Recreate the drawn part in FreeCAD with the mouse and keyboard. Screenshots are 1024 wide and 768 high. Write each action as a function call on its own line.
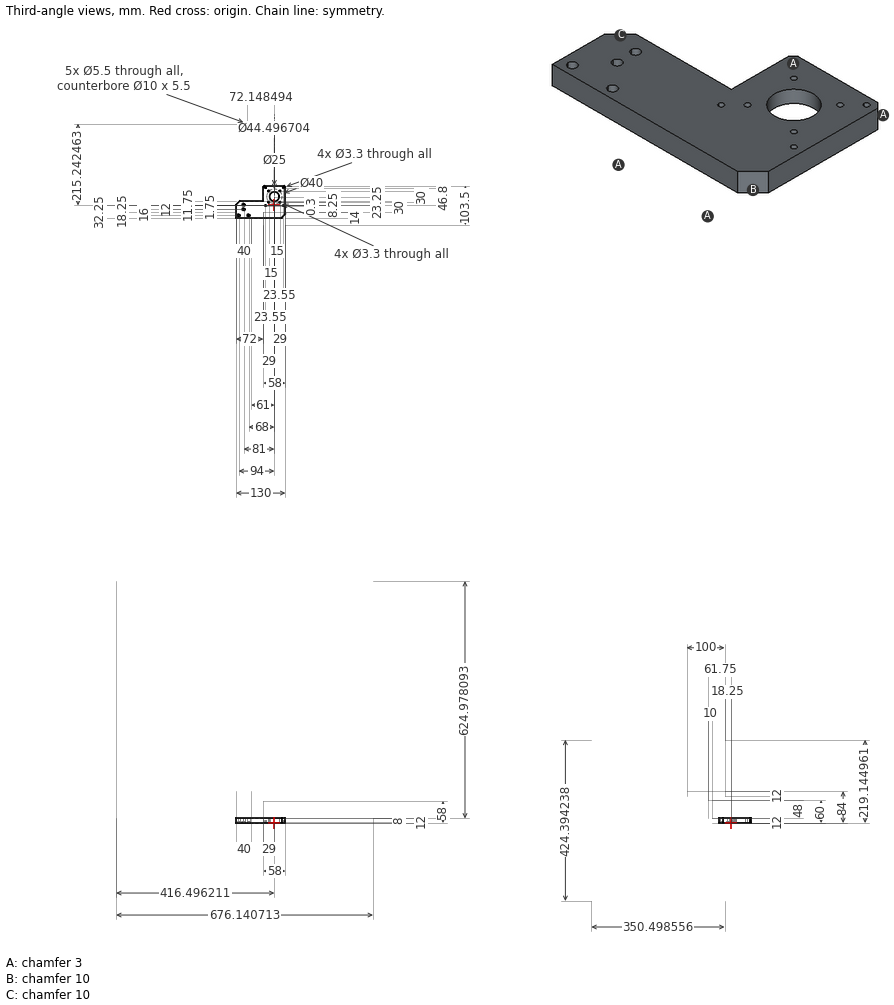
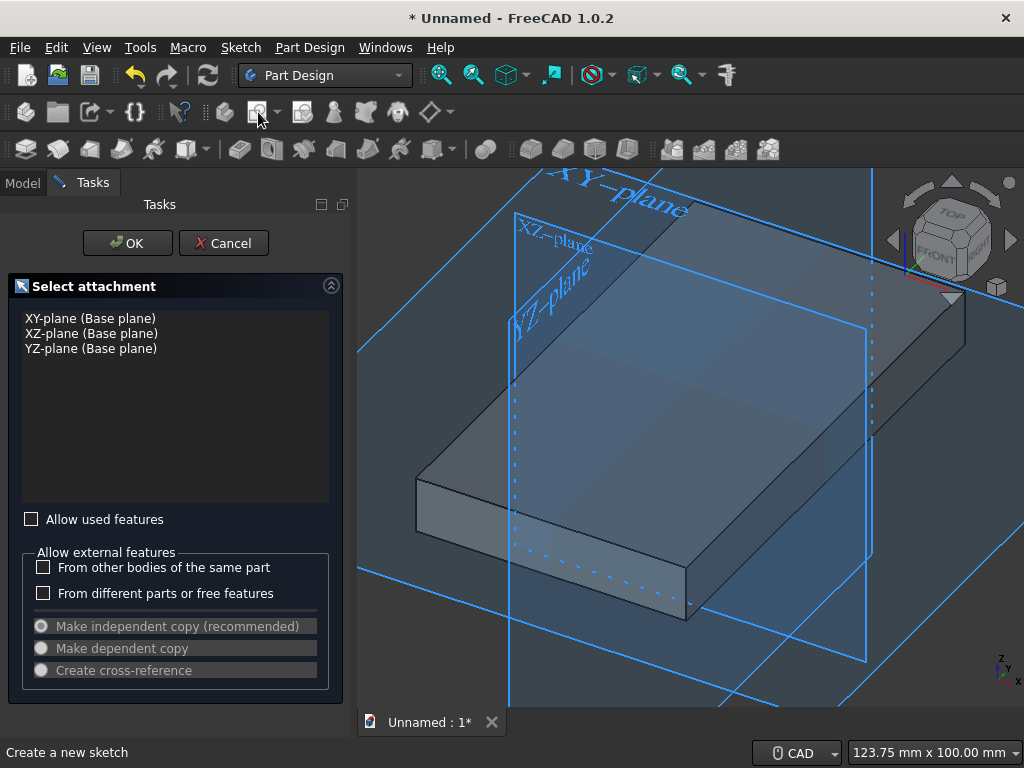
click(82, 318)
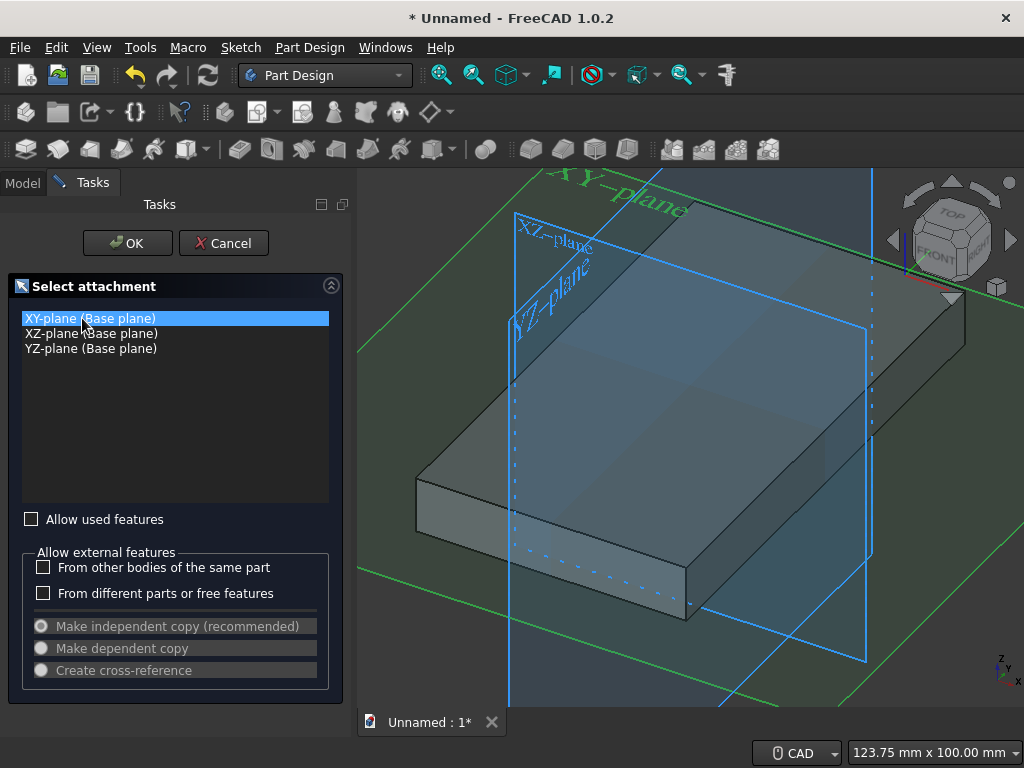
click(128, 243)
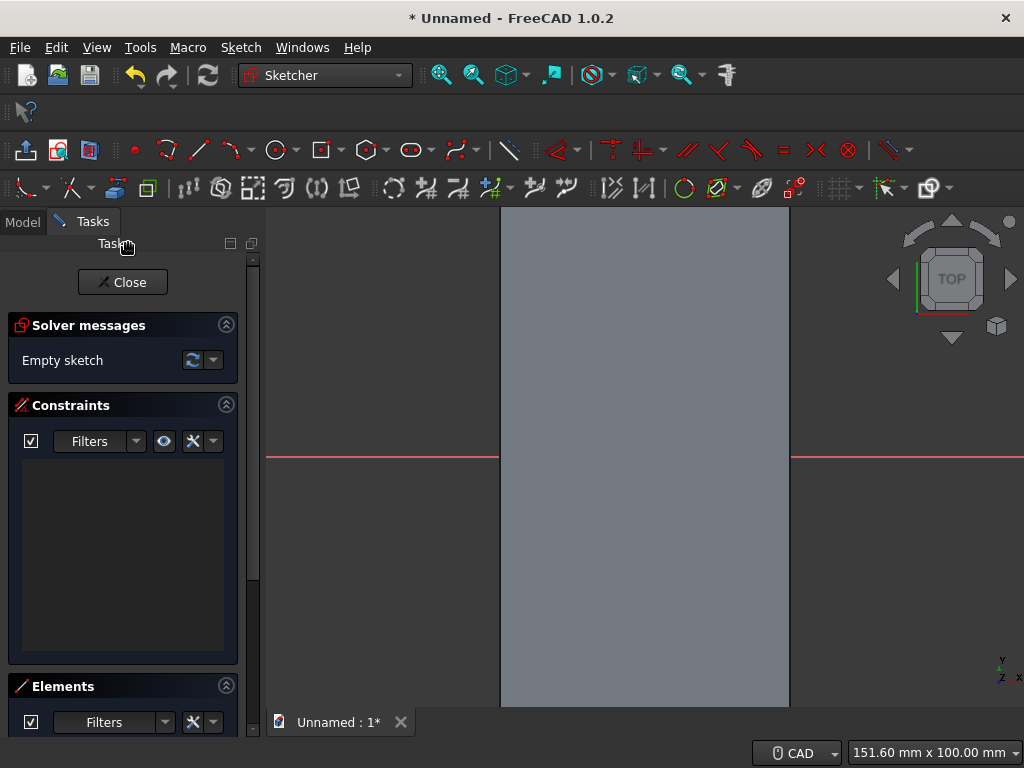
click(90, 150)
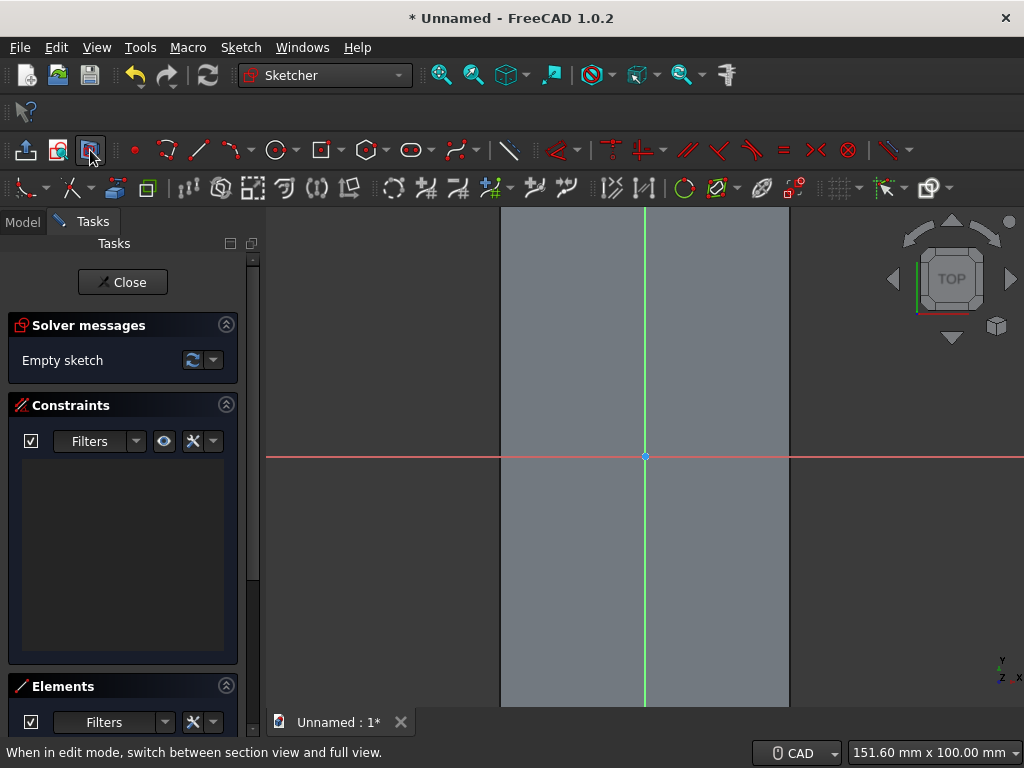
scroll(294, 679, down, 1)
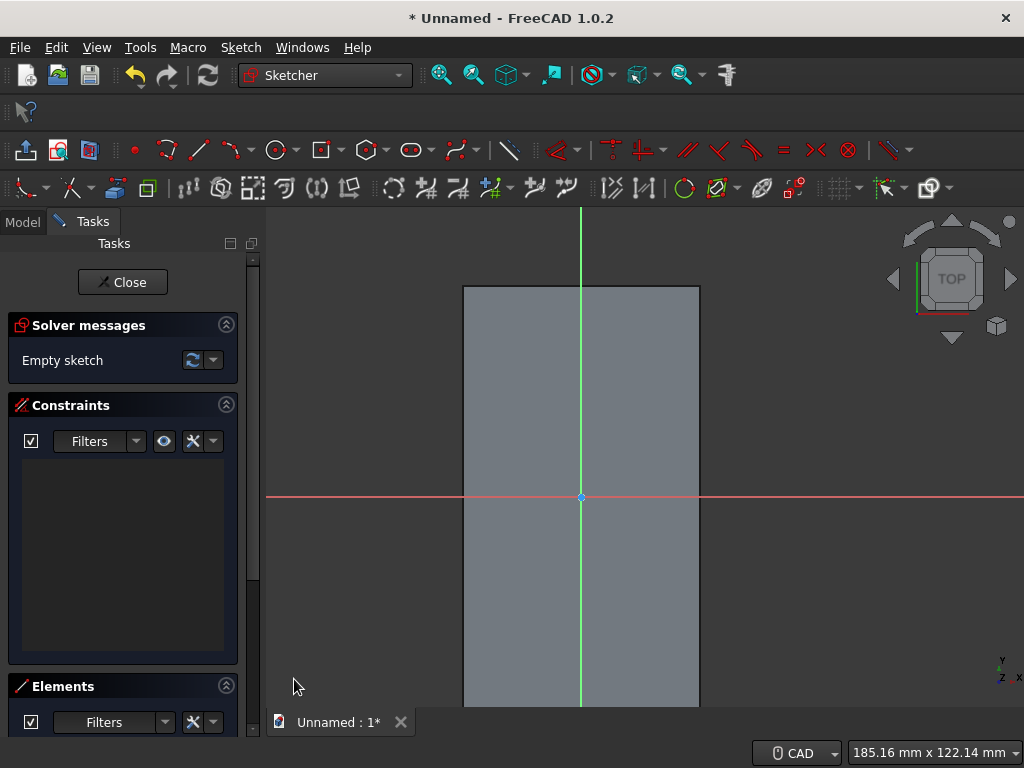
scroll(591, 291, up, 2)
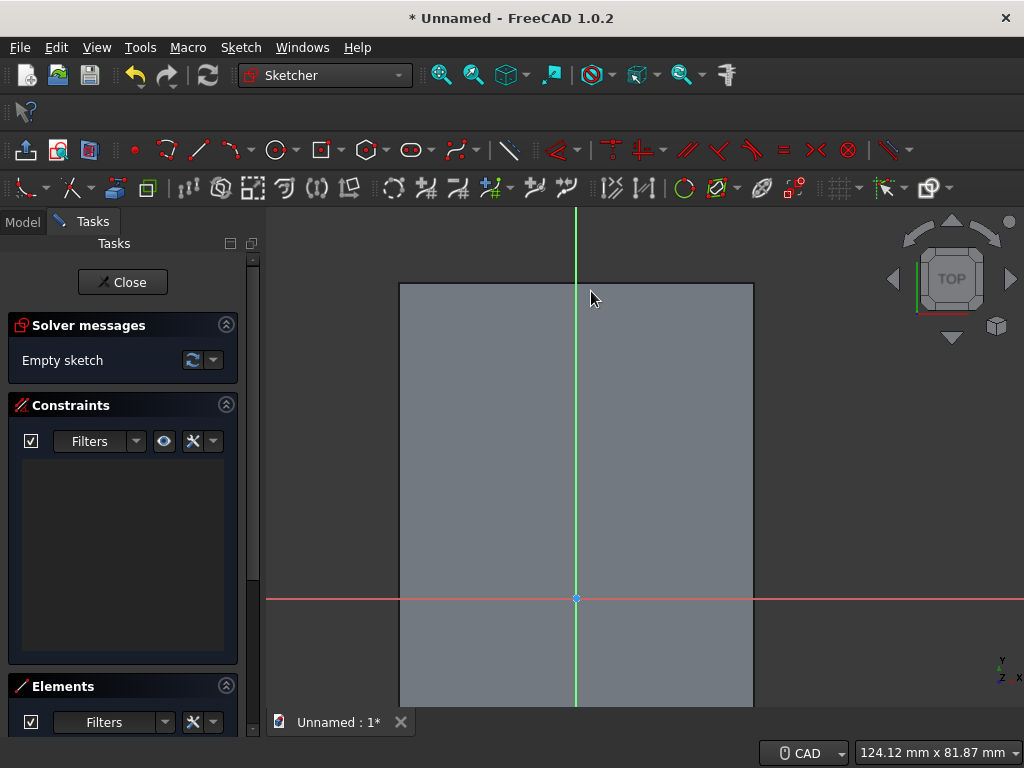
click(276, 150)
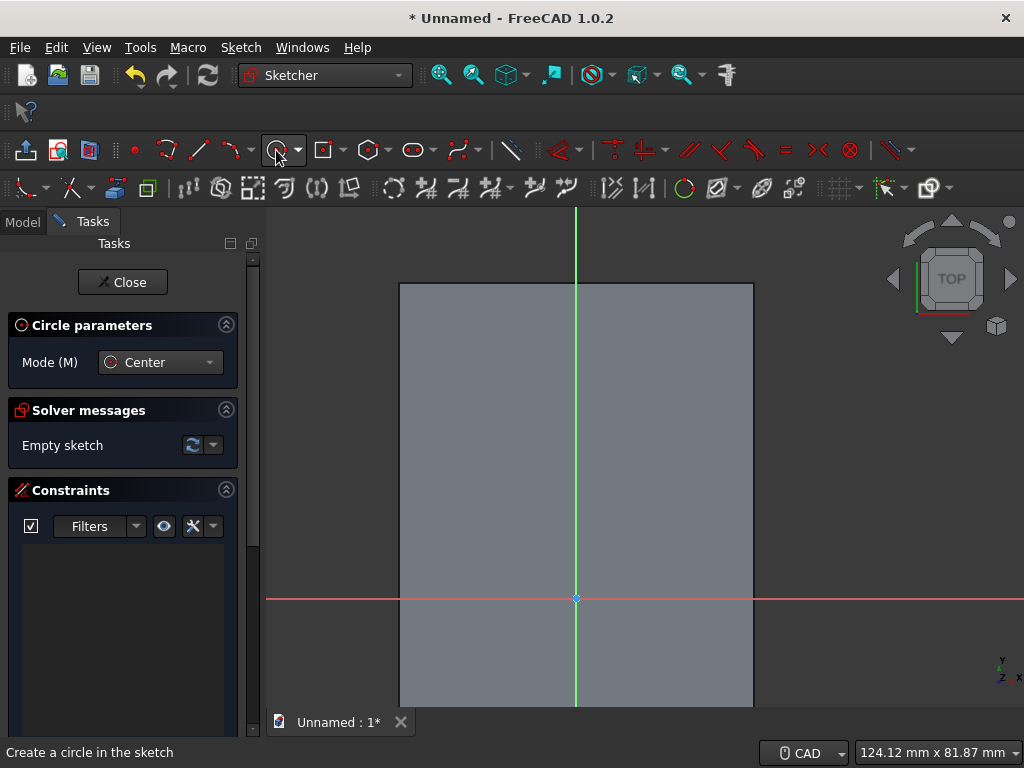
scroll(720, 313, up, 5)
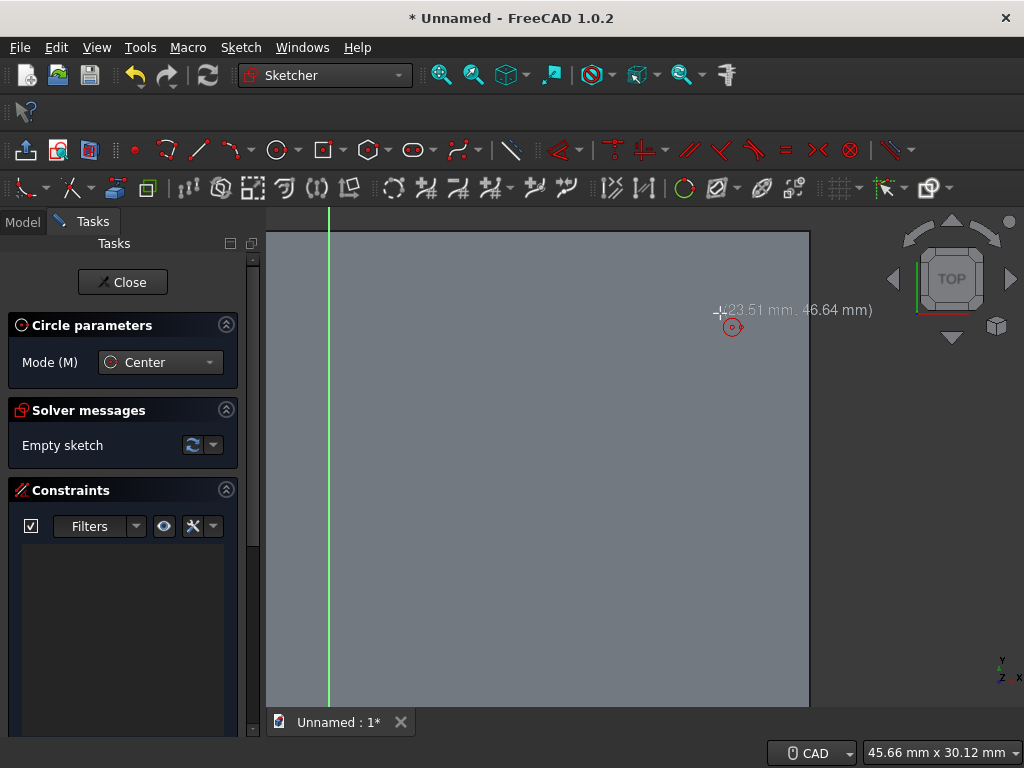
click(720, 313)
move(739, 293)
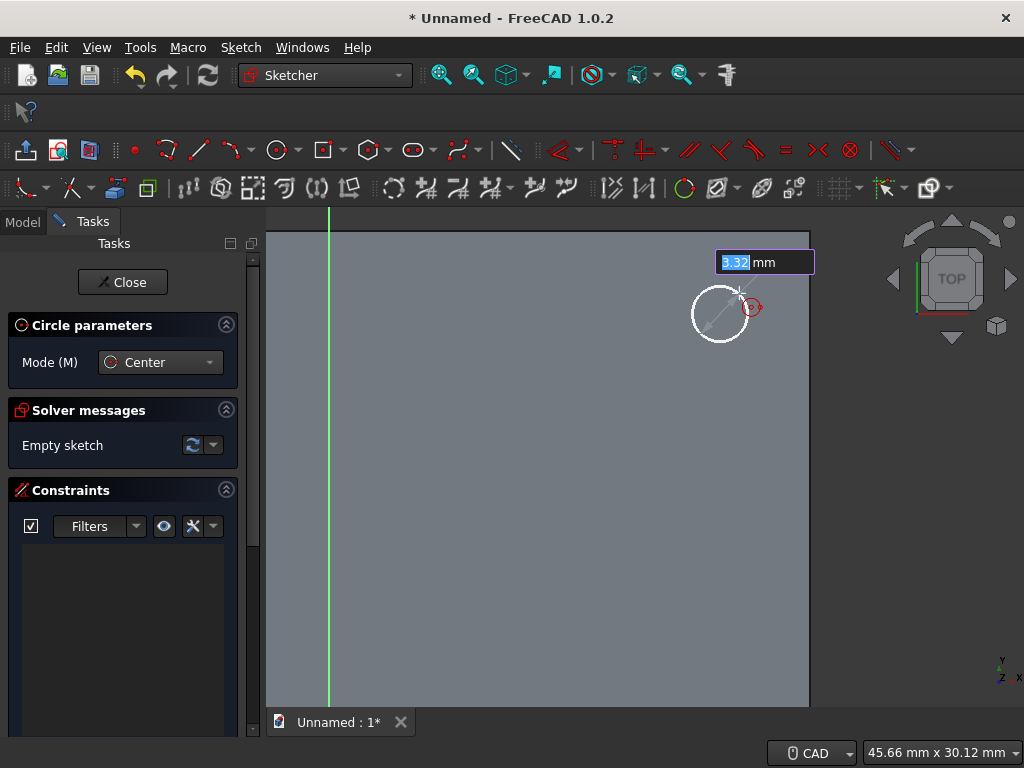
text(3.3)
key(Return)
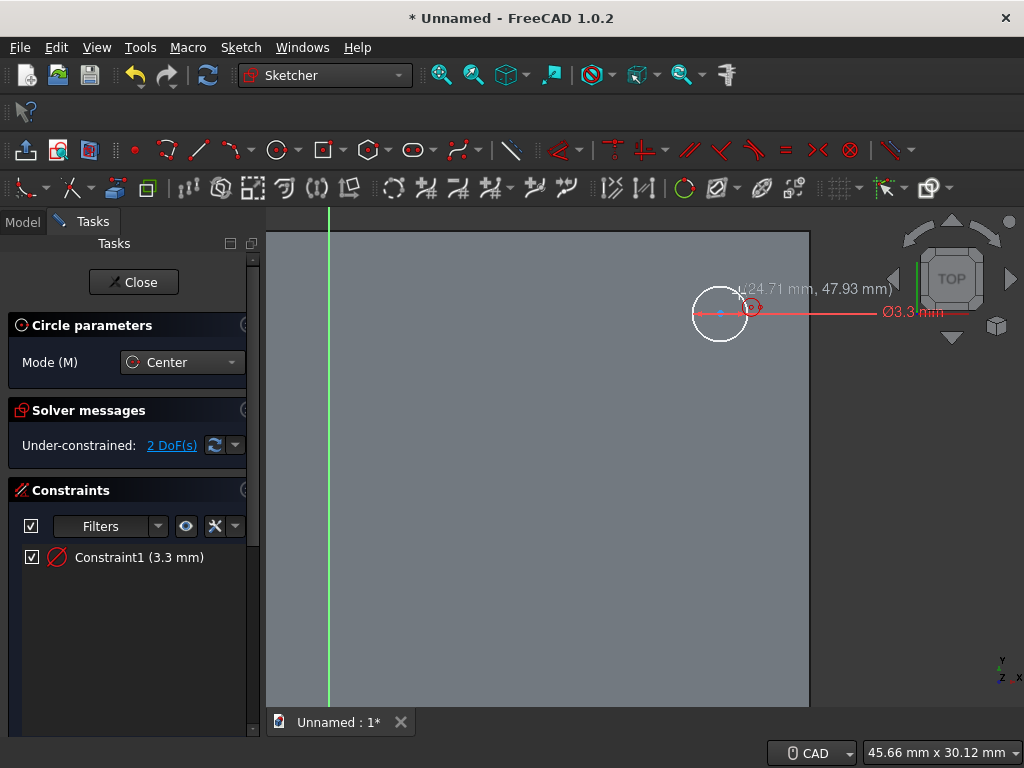
scroll(721, 313, down, 5)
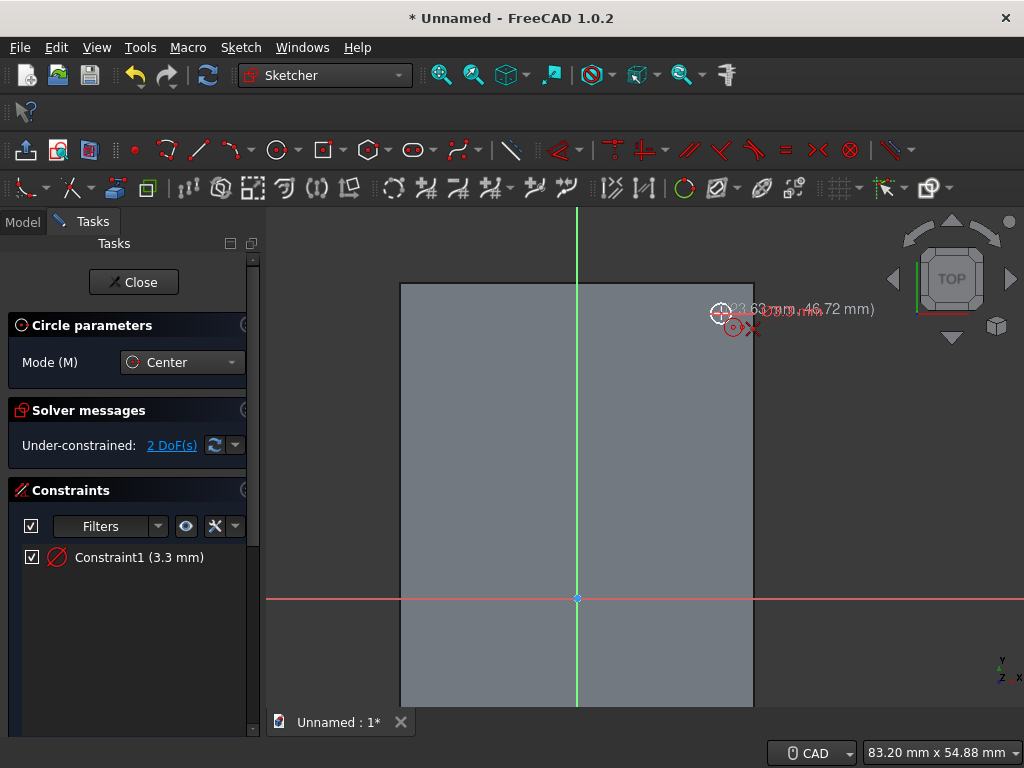
scroll(433, 313, up, 5)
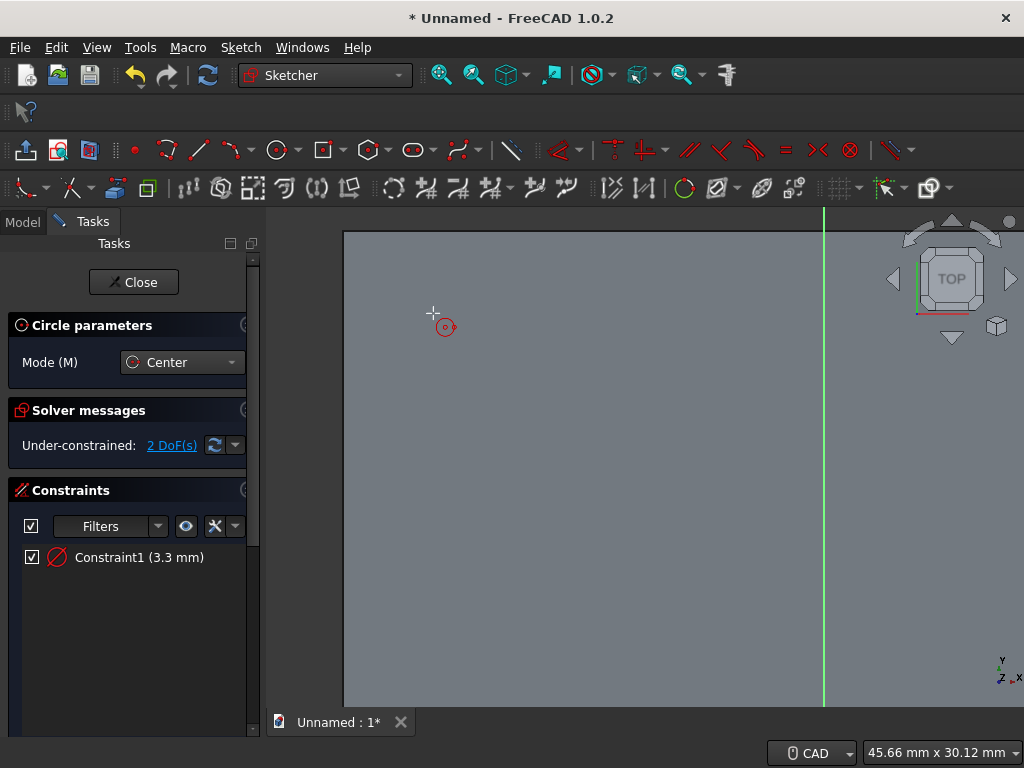
click(433, 313)
move(453, 293)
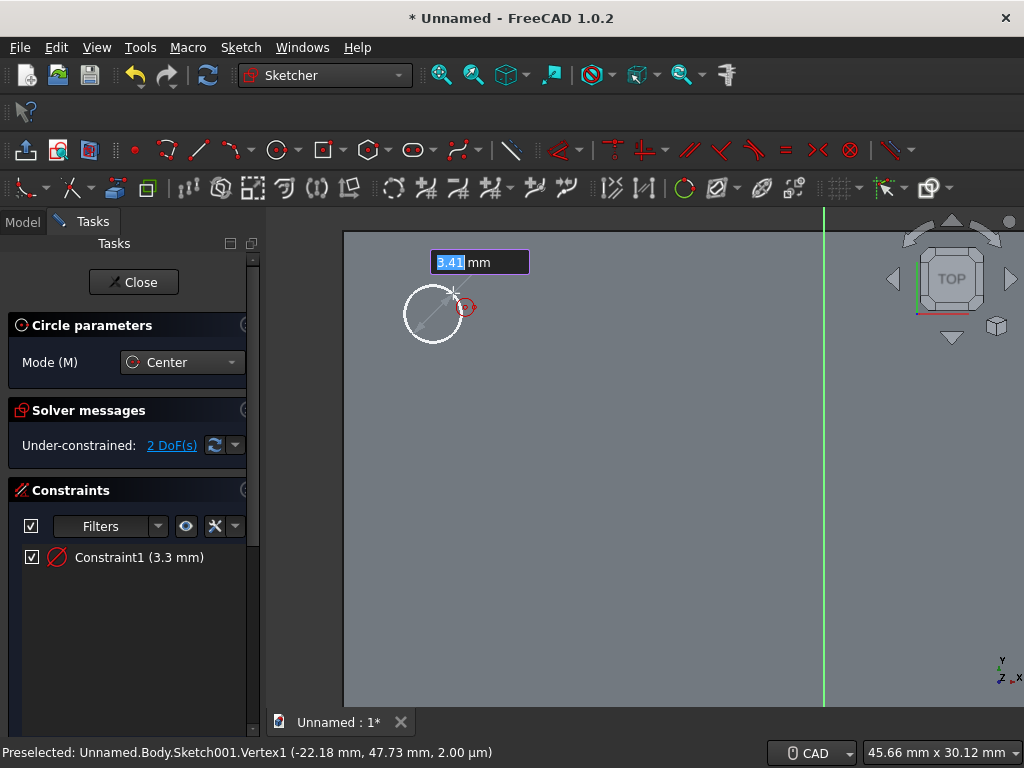
text(3.3)
key(Return)